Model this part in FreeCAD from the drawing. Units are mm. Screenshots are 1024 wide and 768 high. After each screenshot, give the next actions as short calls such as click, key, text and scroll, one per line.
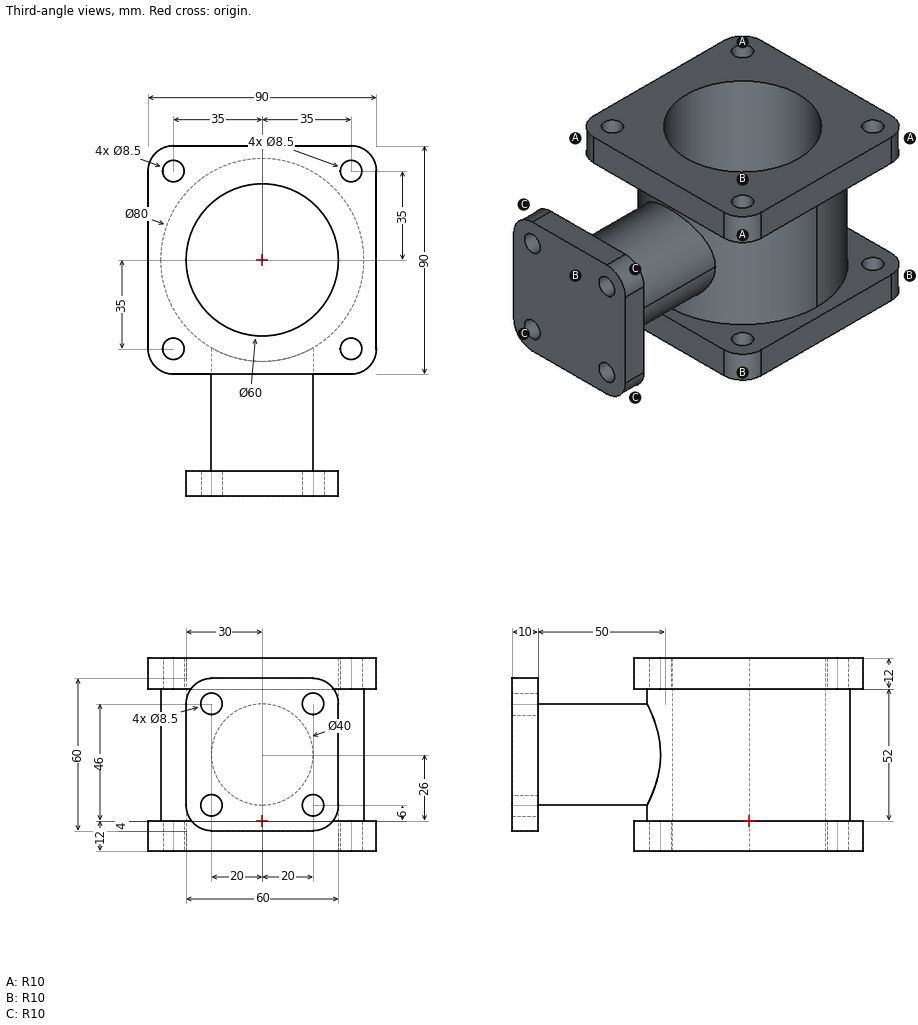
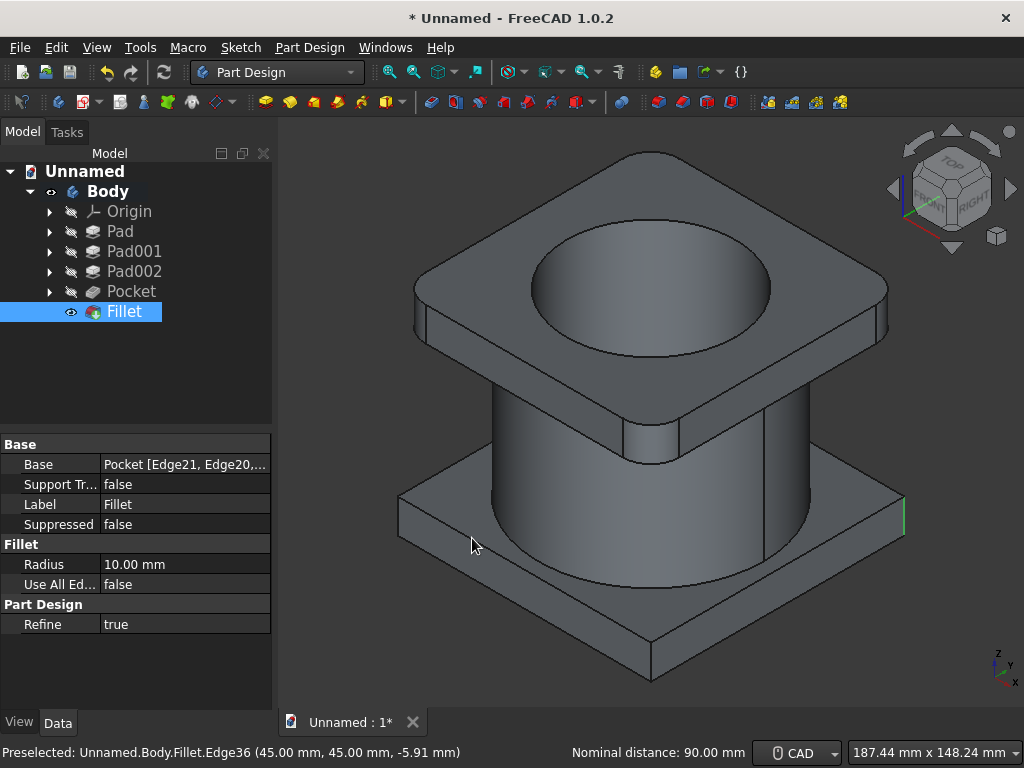
click(651, 661, ctrl)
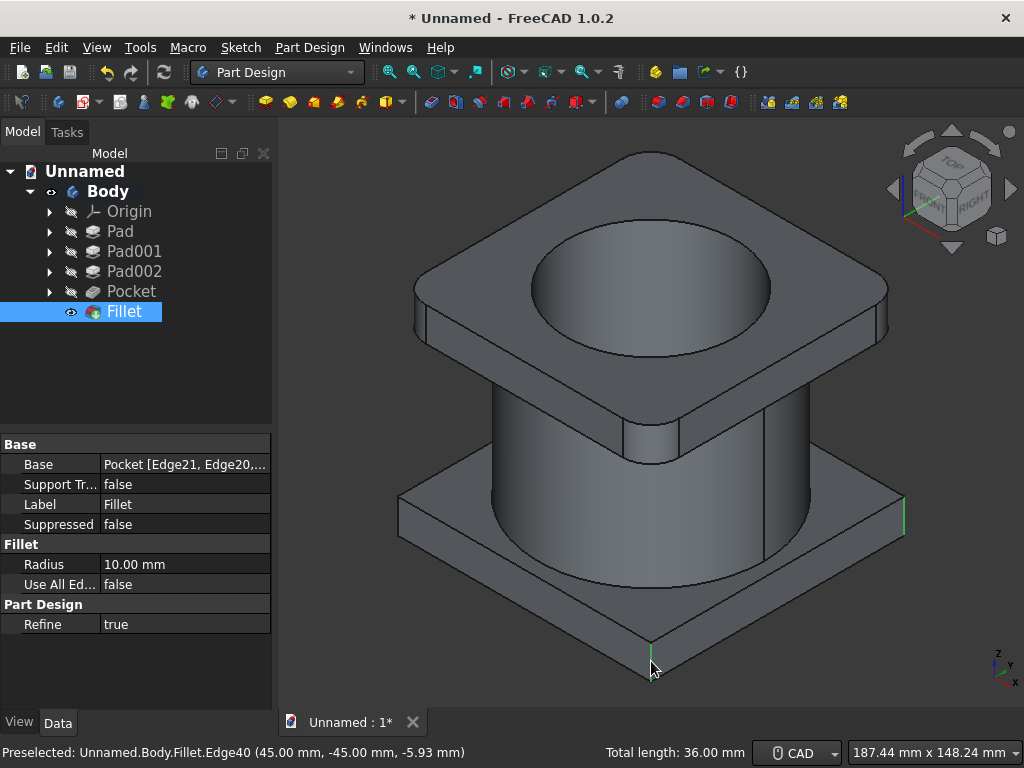
key(2)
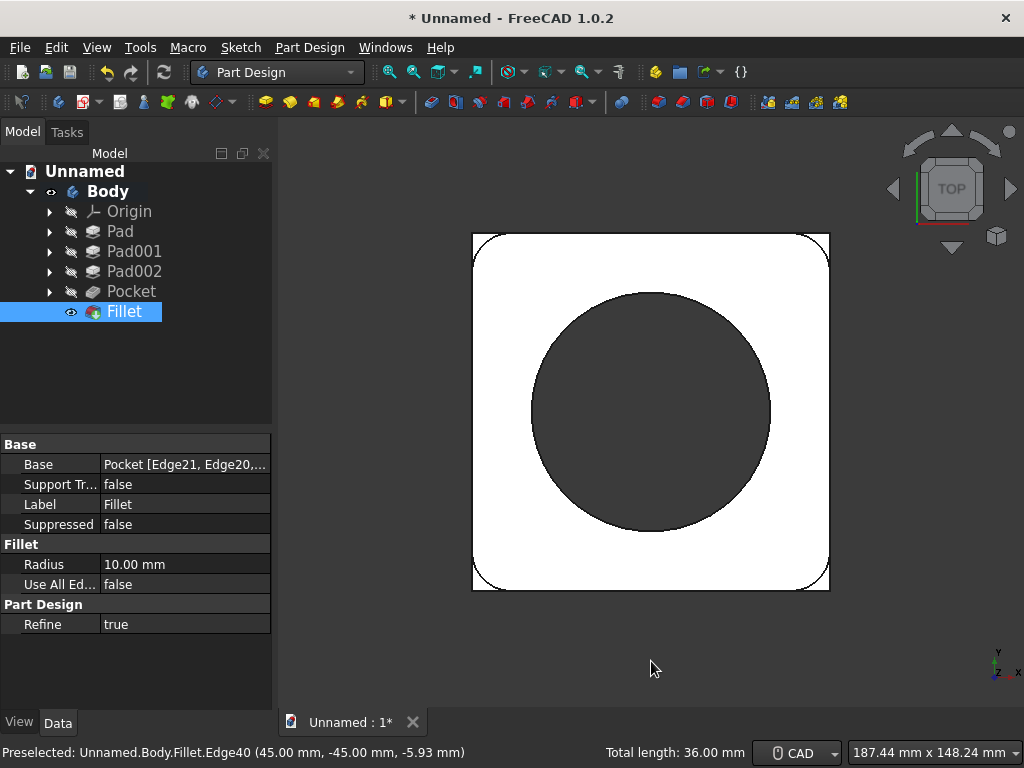
key(1)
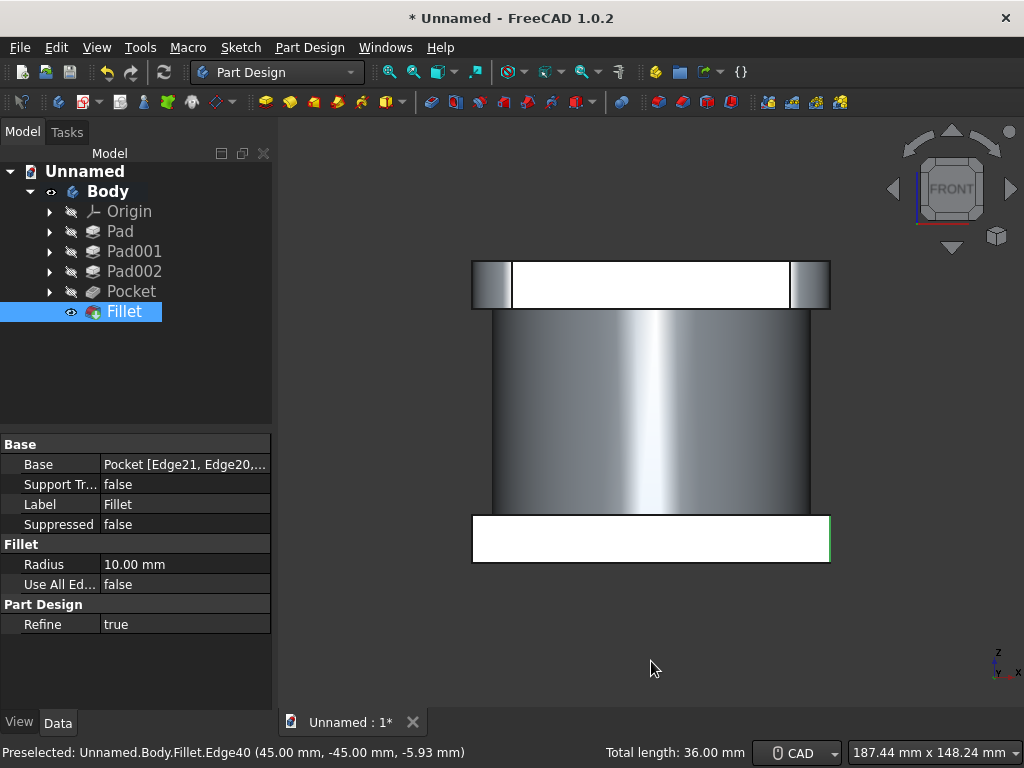
click(472, 538, ctrl)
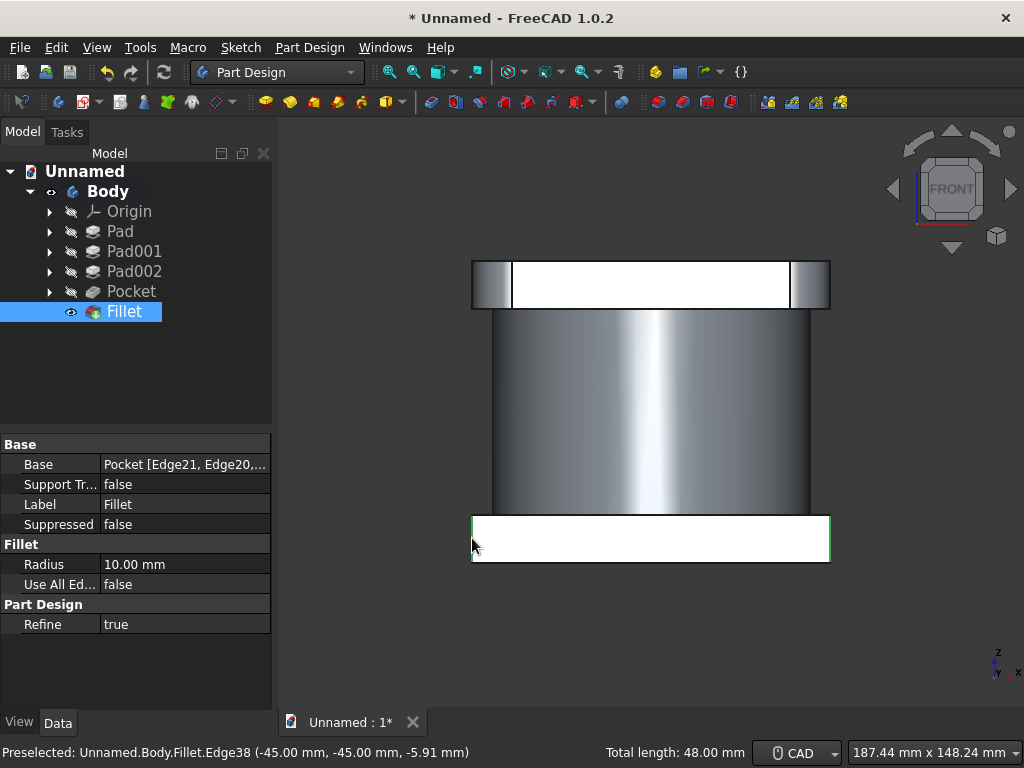
click(660, 102)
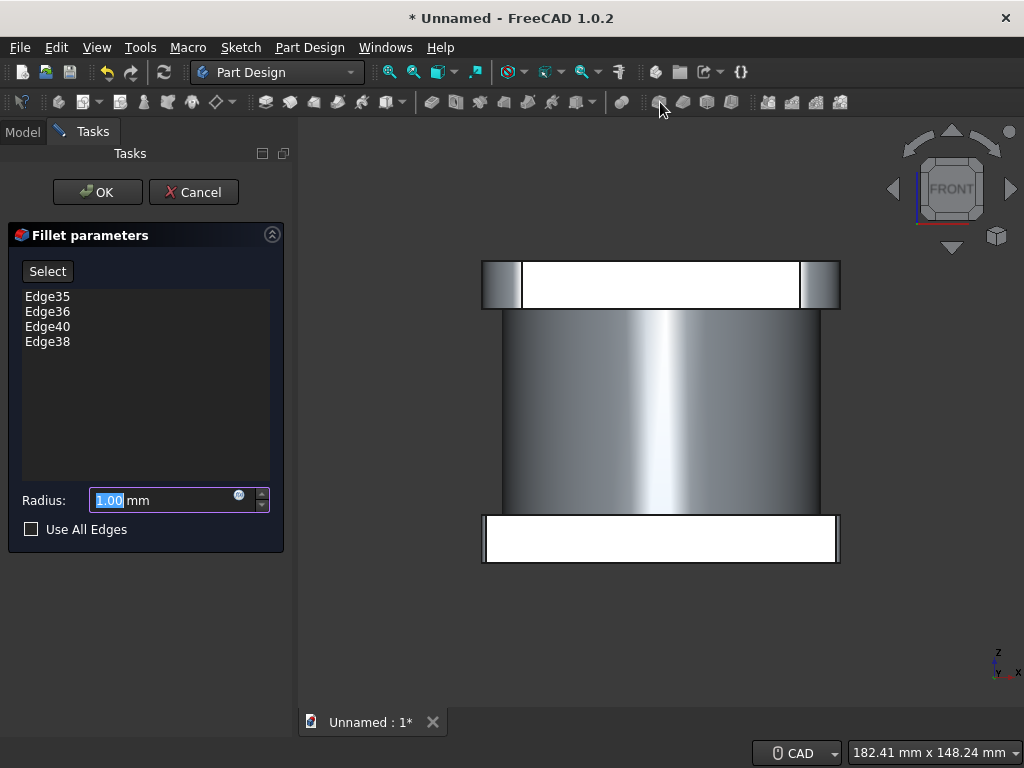
text(10)
key(Tab)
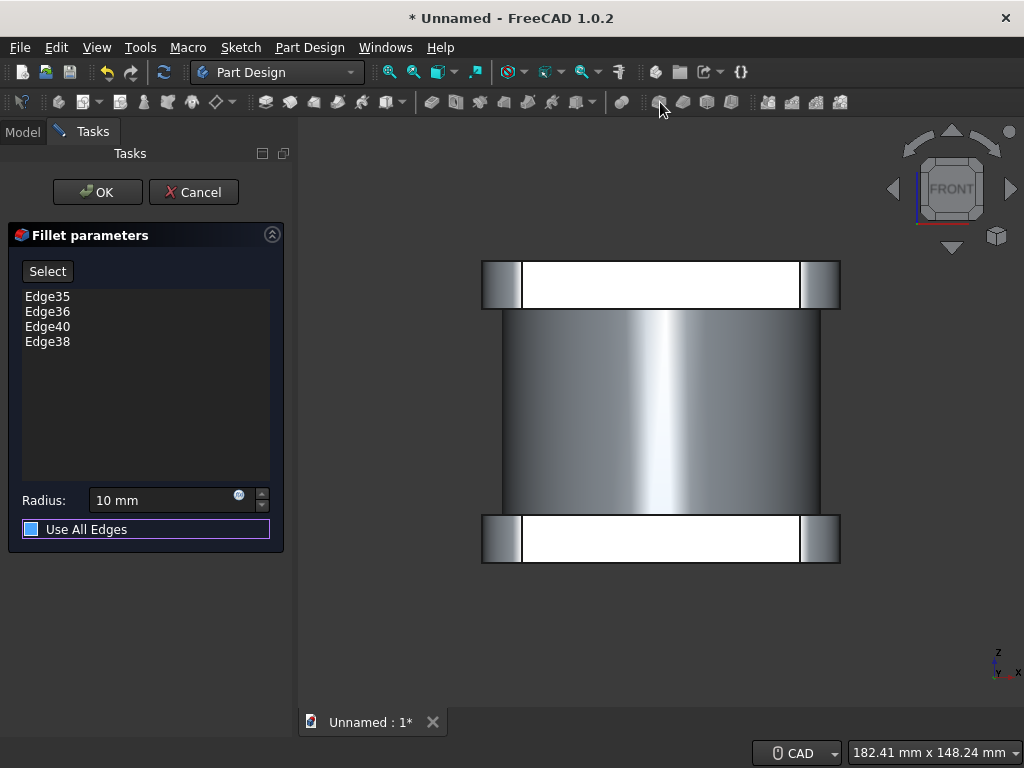
click(98, 192)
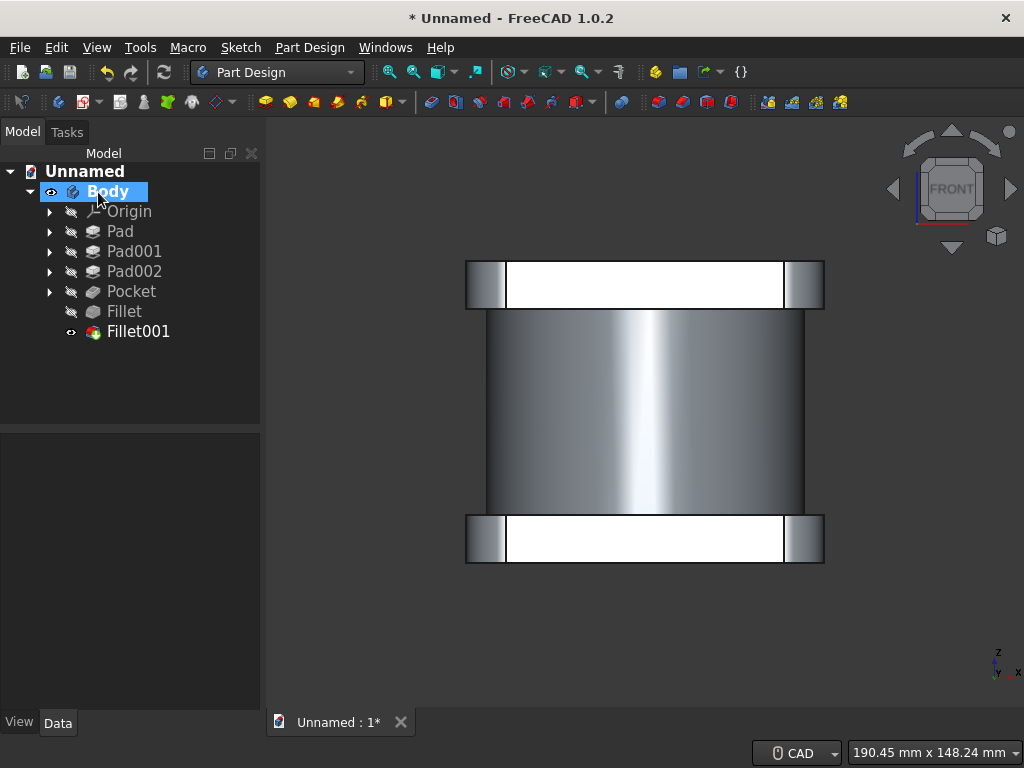
key(5)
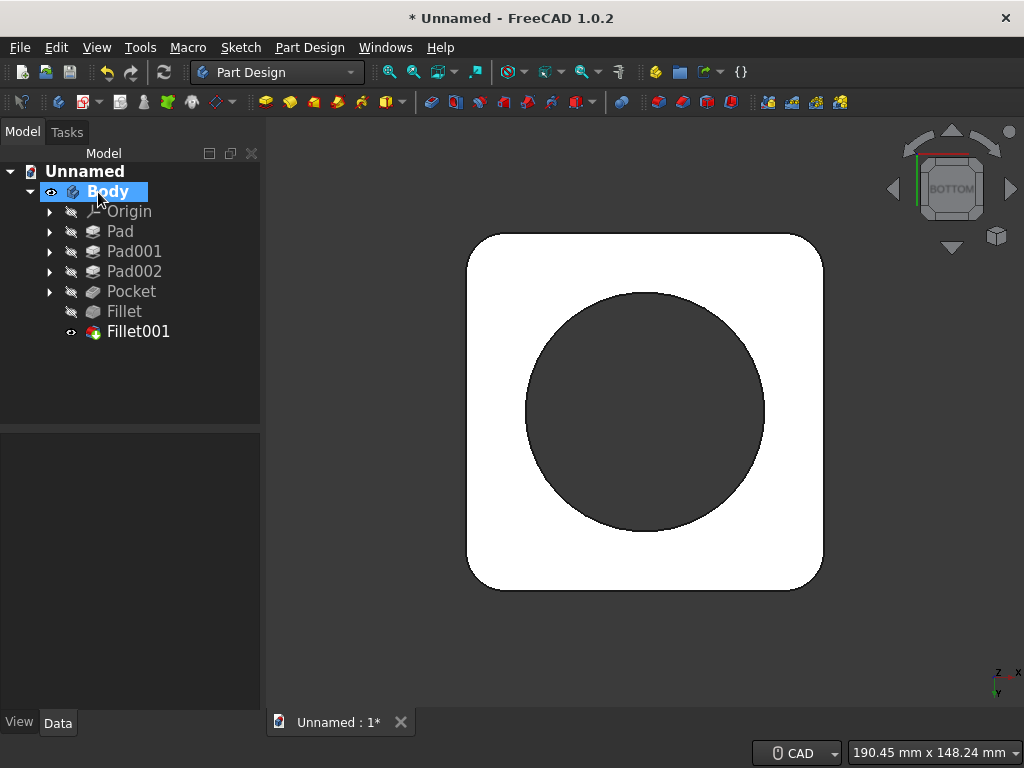
click(799, 513)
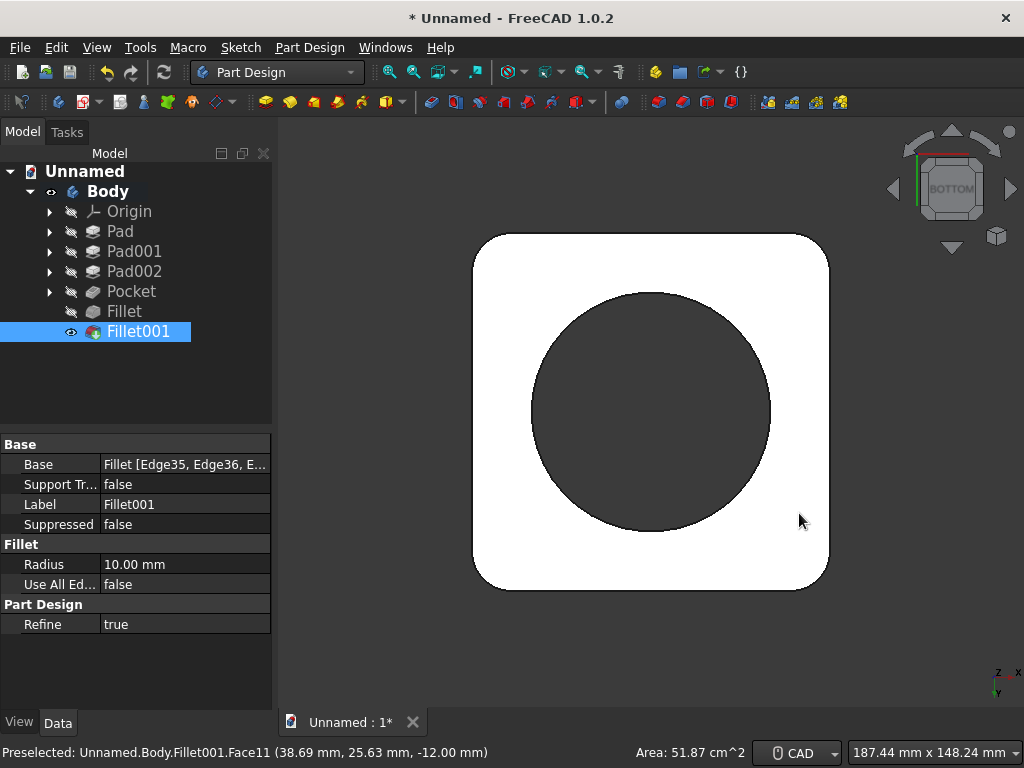
click(84, 102)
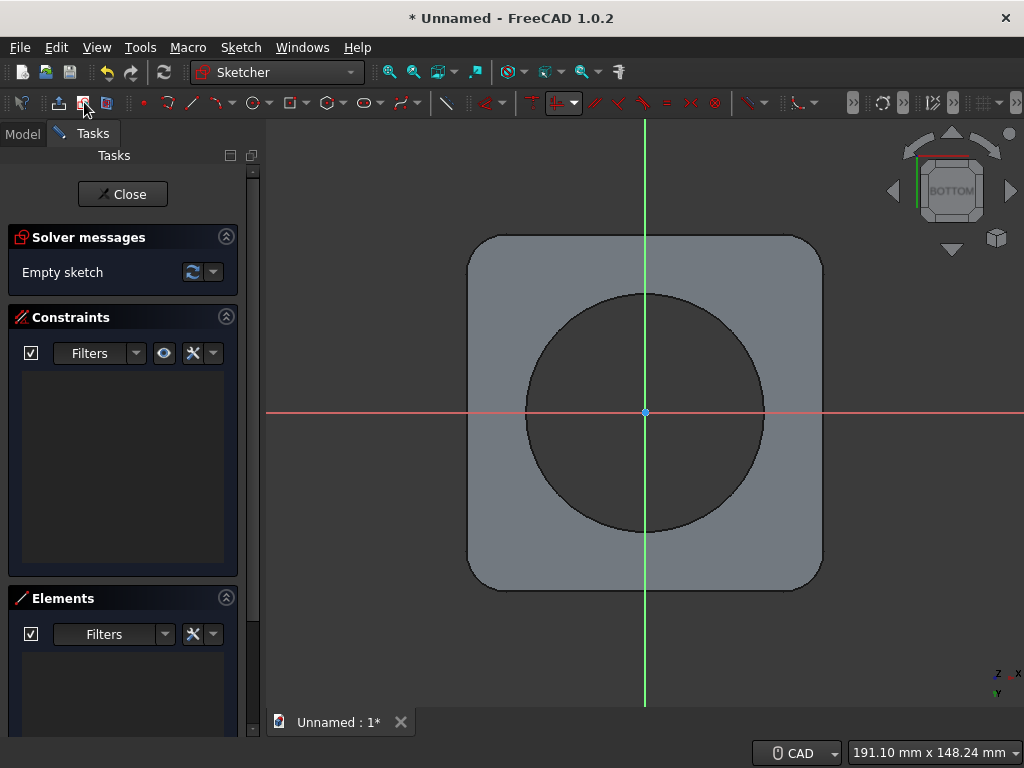
click(254, 104)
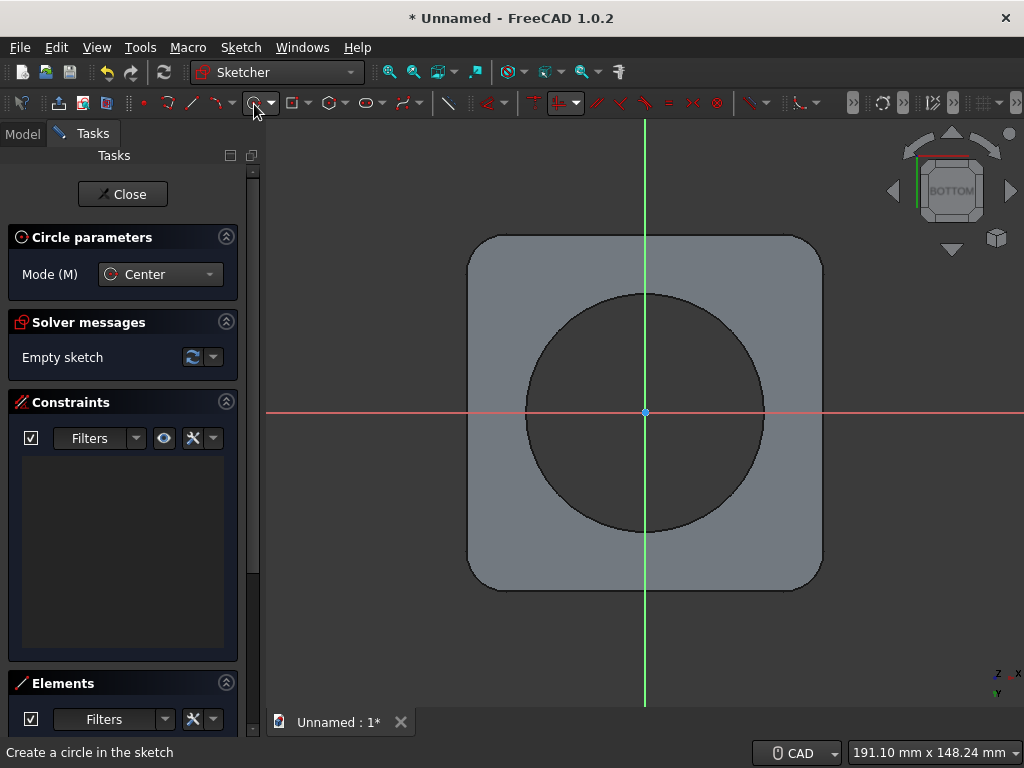
scroll(784, 552, up, 2)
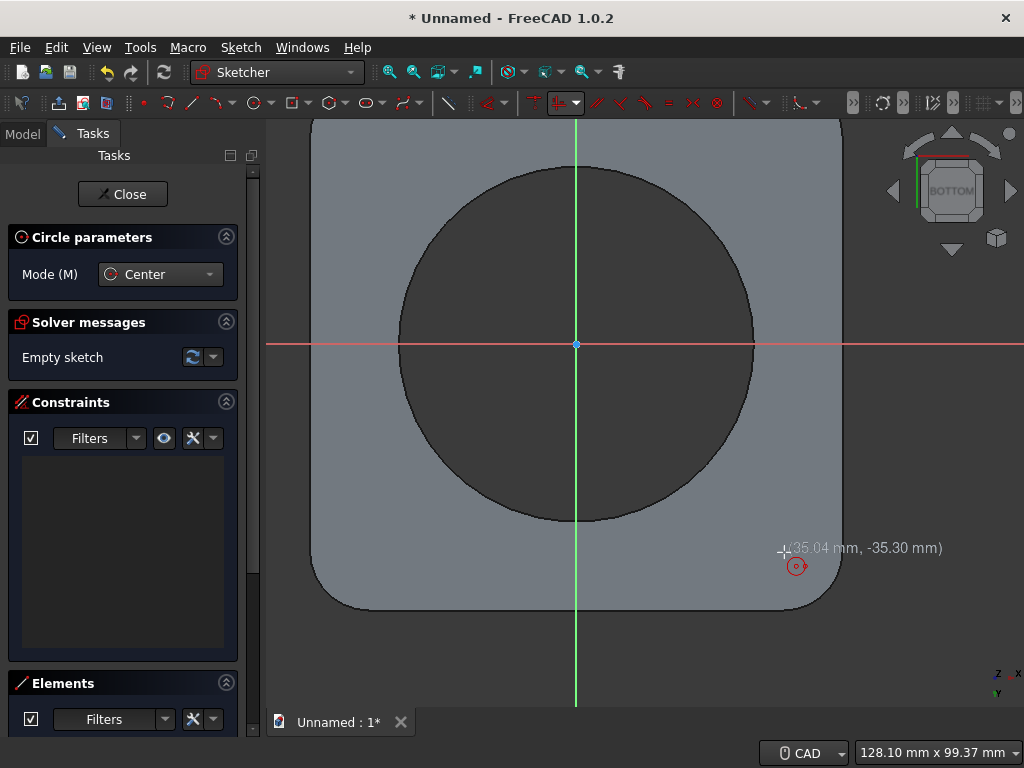
click(783, 551)
click(801, 534)